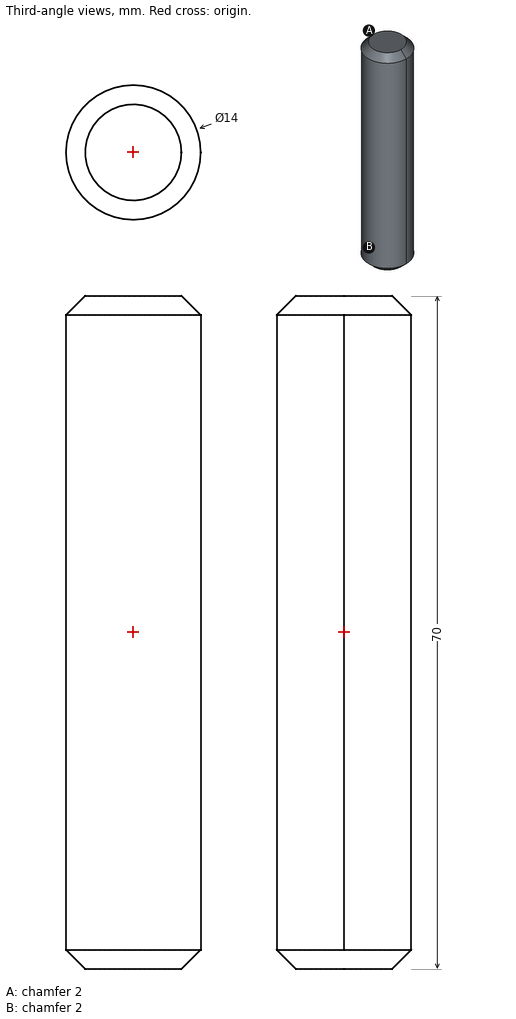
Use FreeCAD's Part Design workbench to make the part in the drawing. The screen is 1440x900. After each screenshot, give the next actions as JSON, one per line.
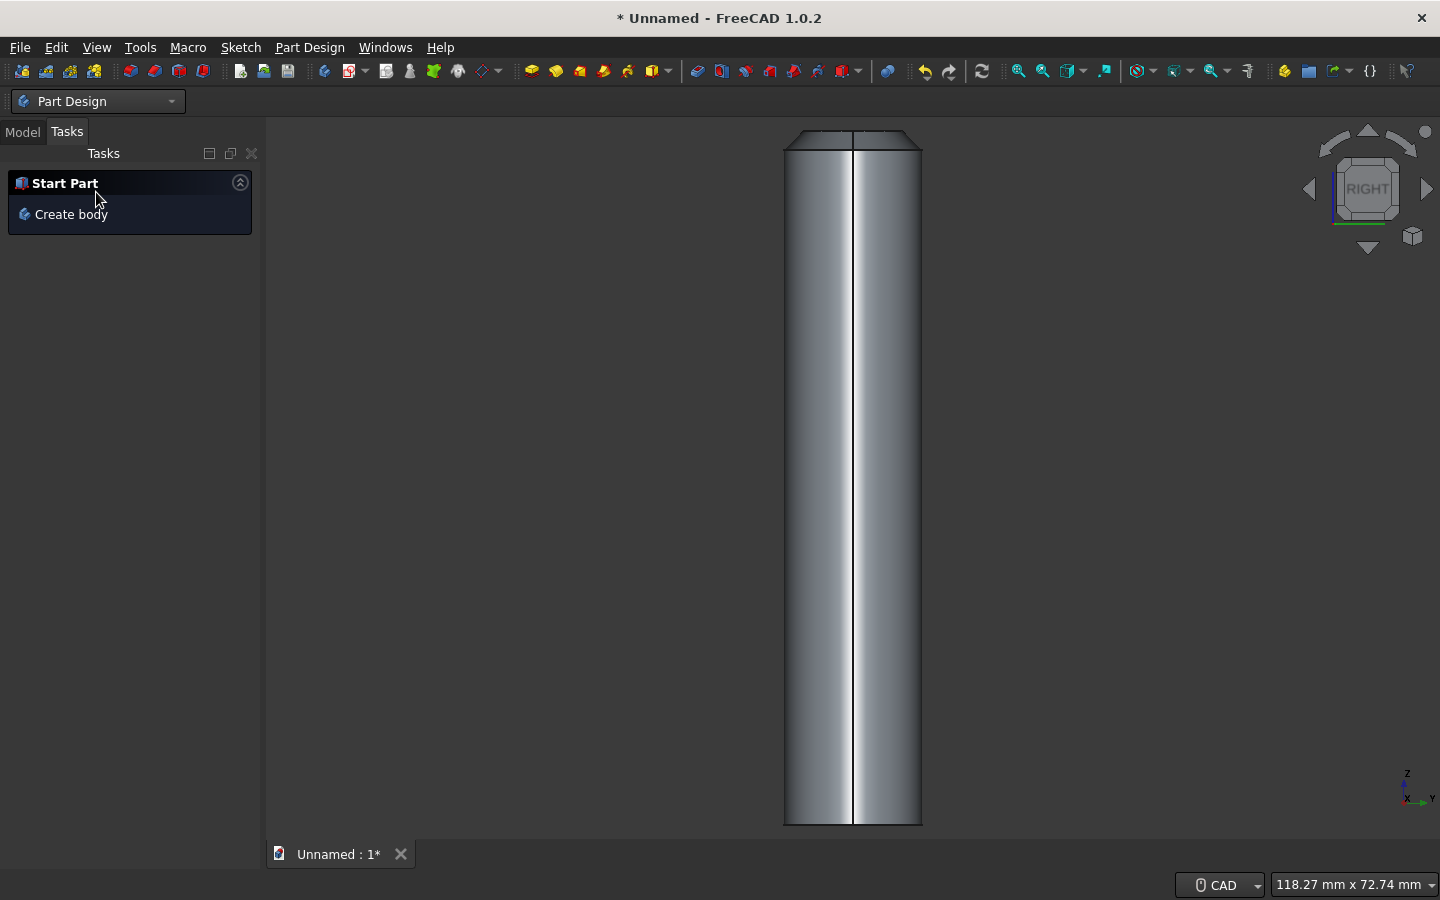
{"action": "key", "text": "5"}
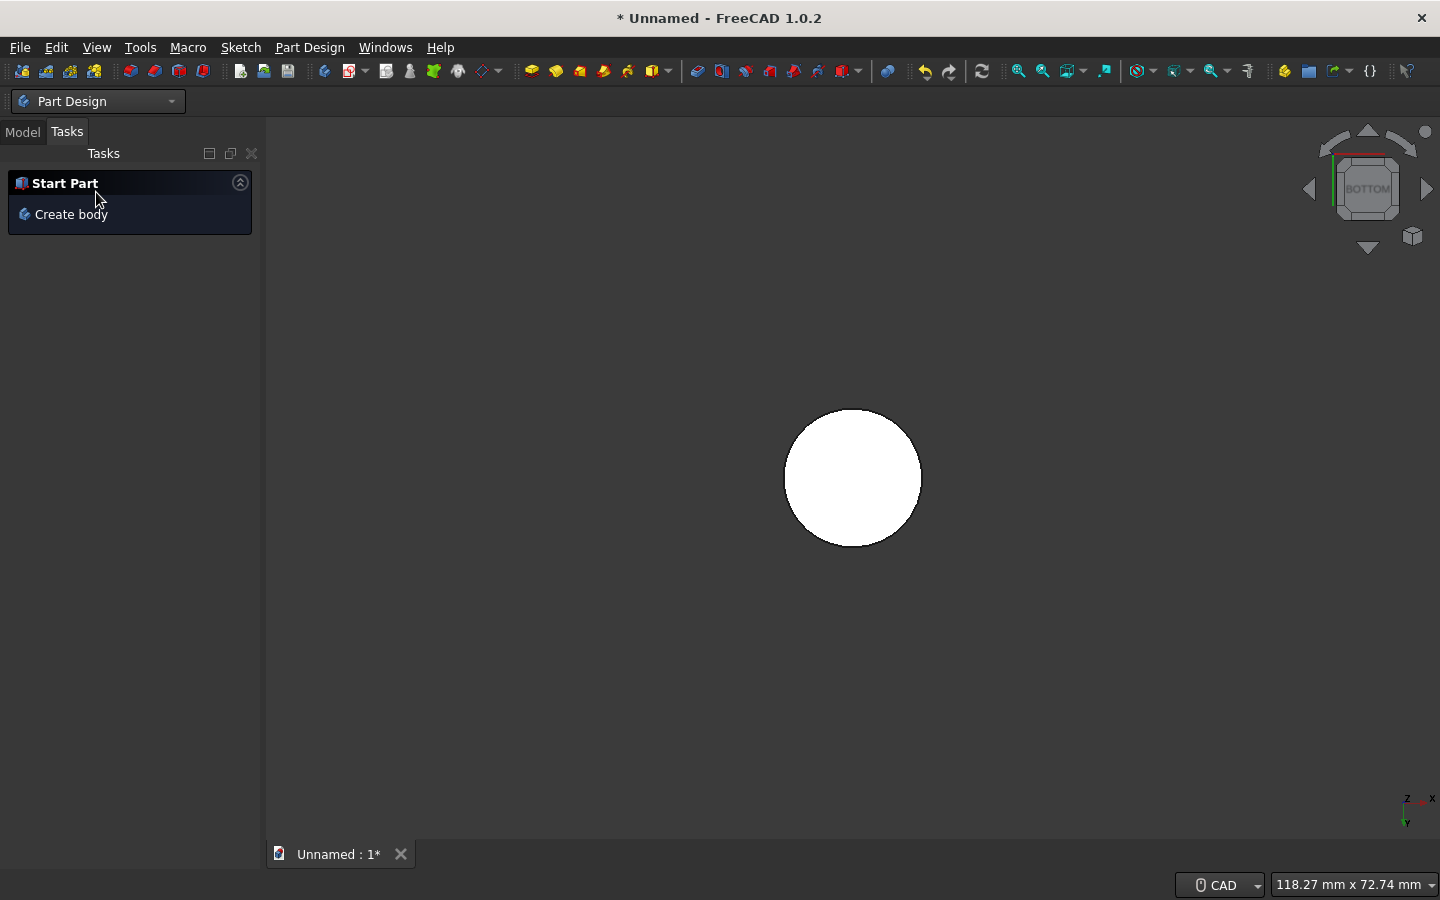
{"action": "key", "text": "v f"}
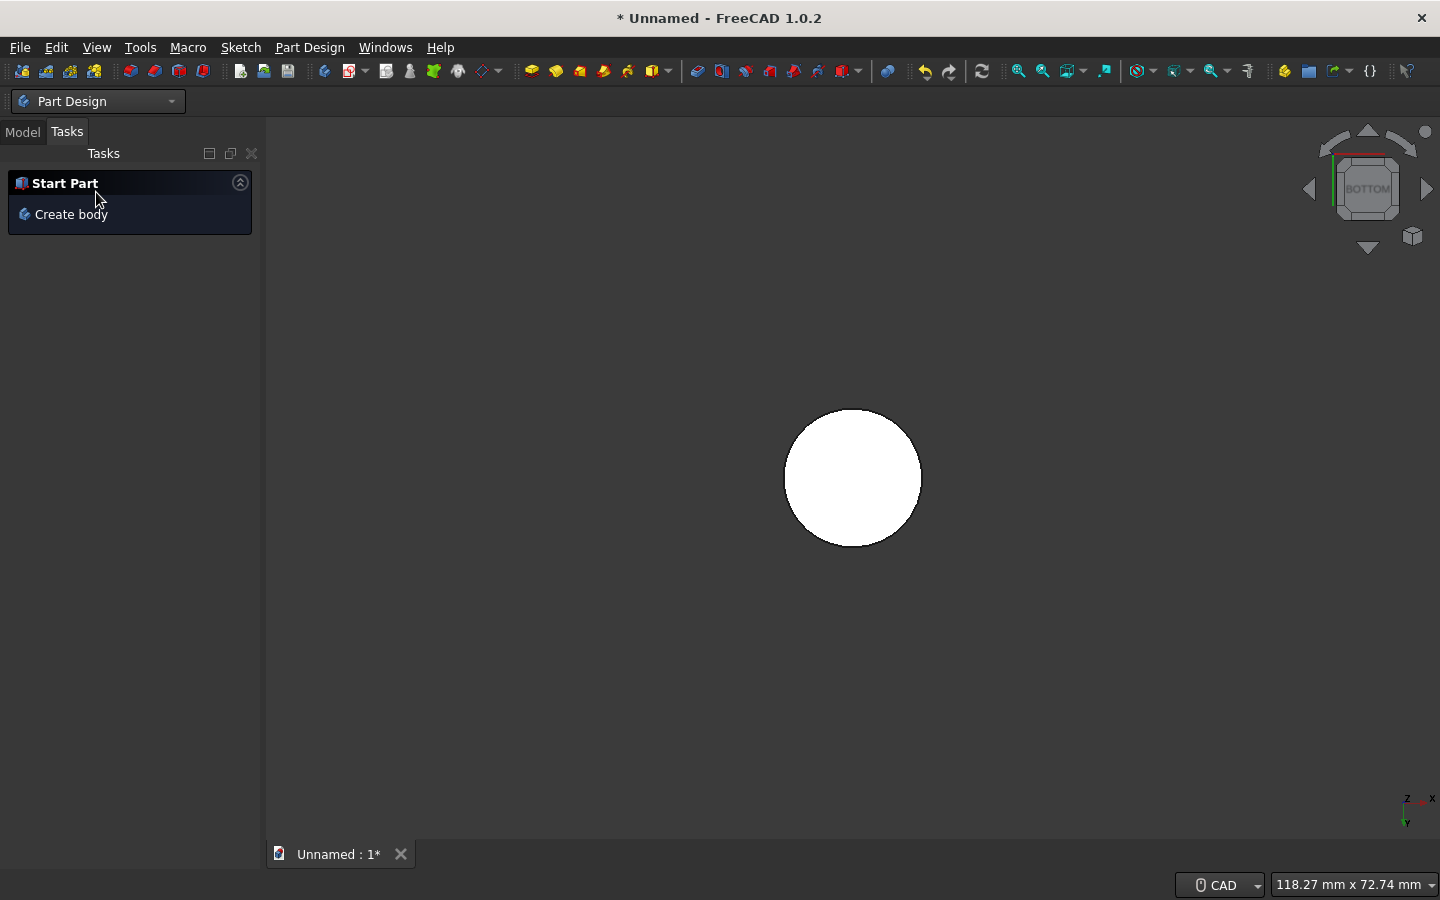
{"action": "left_click", "coordinate": [783, 477]}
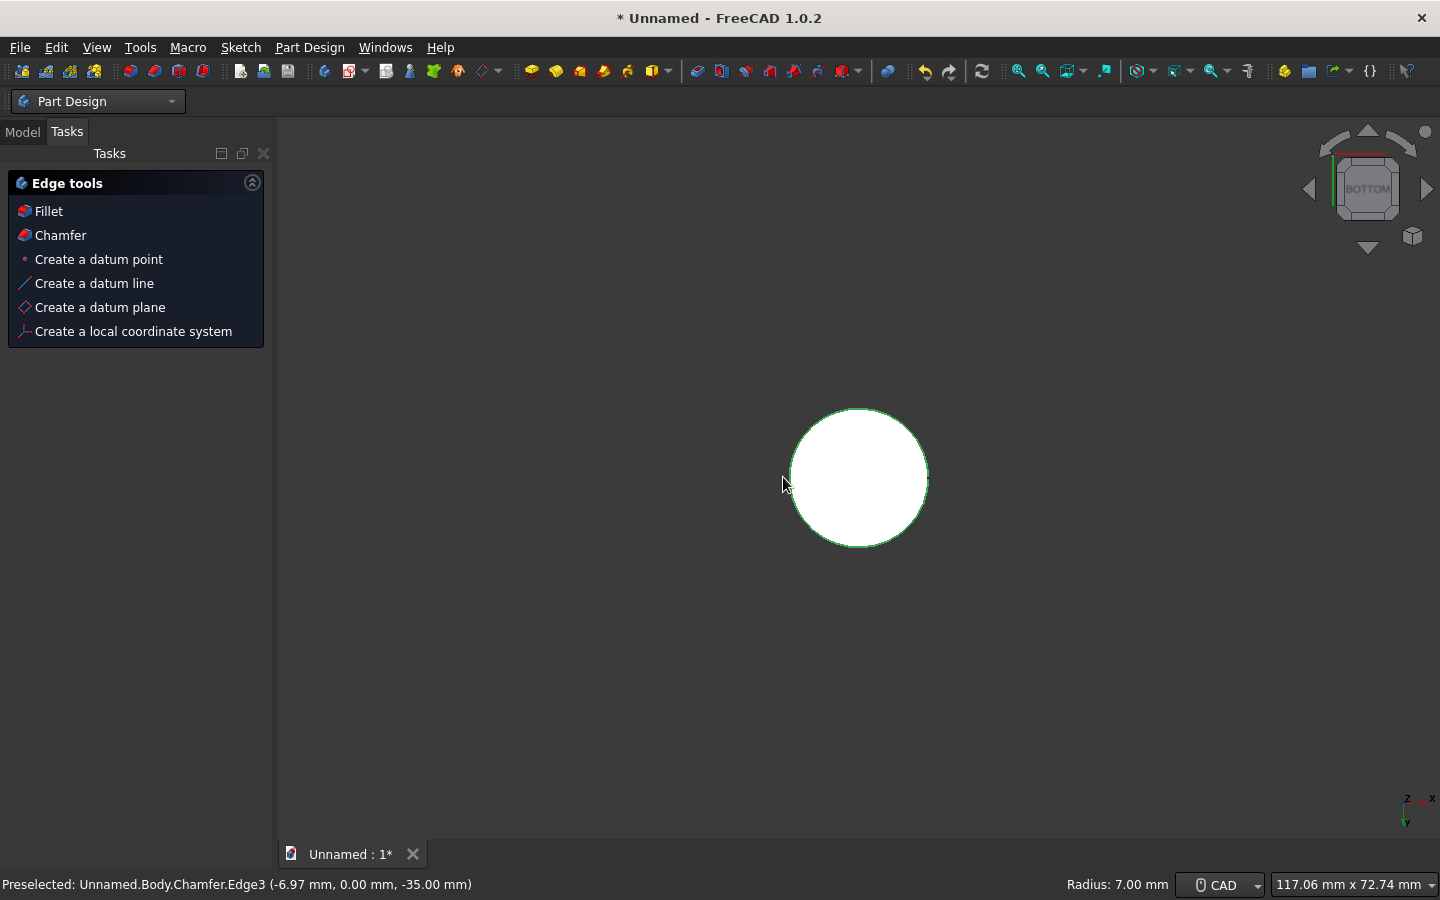
{"action": "left_click", "coordinate": [156, 72]}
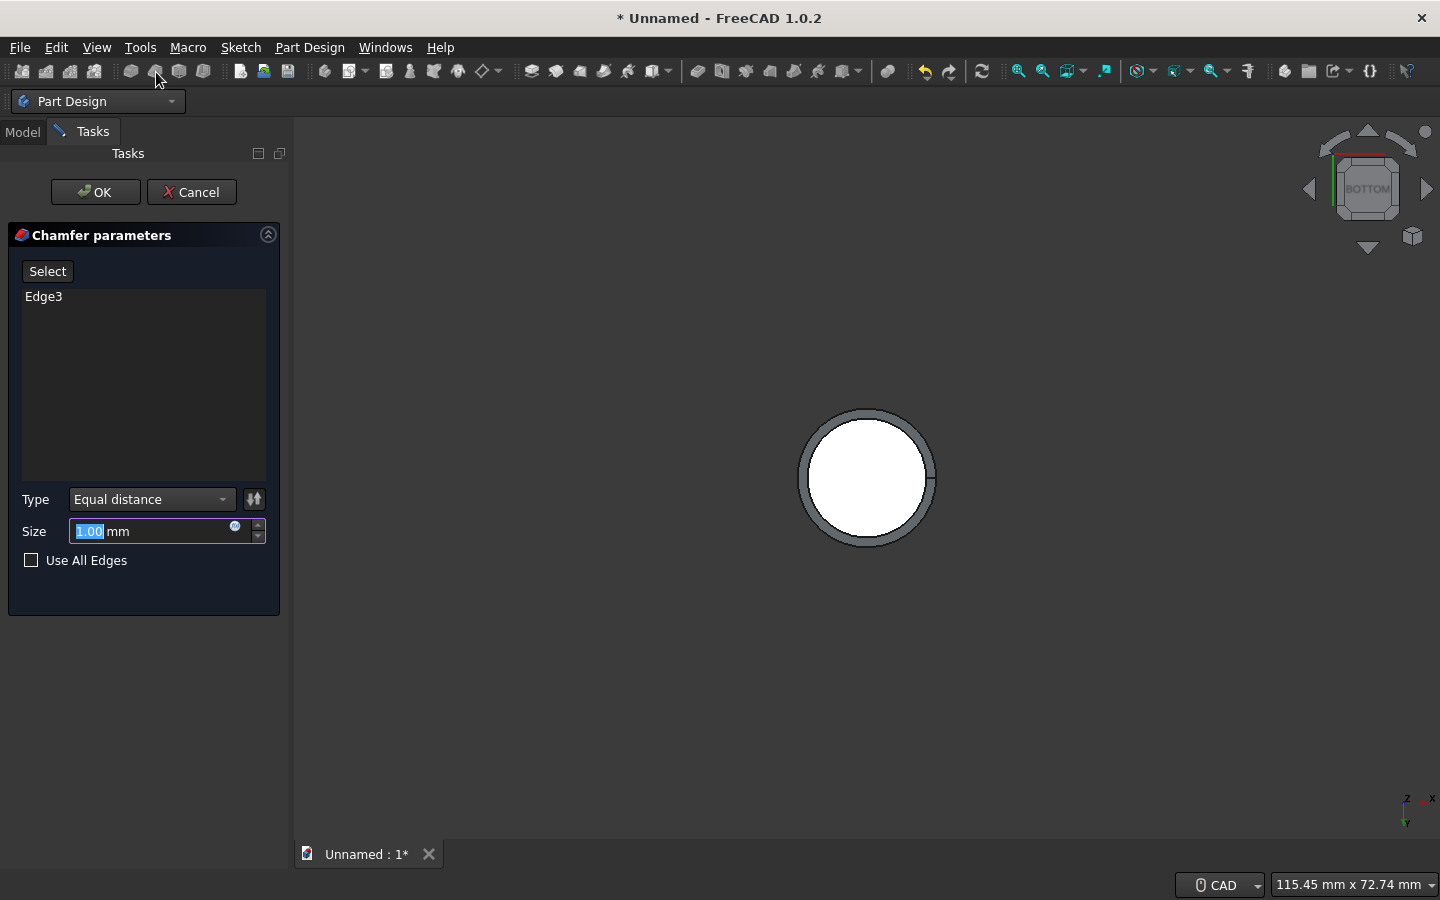
{"action": "type", "text": "2"}
{"action": "key", "text": "Tab"}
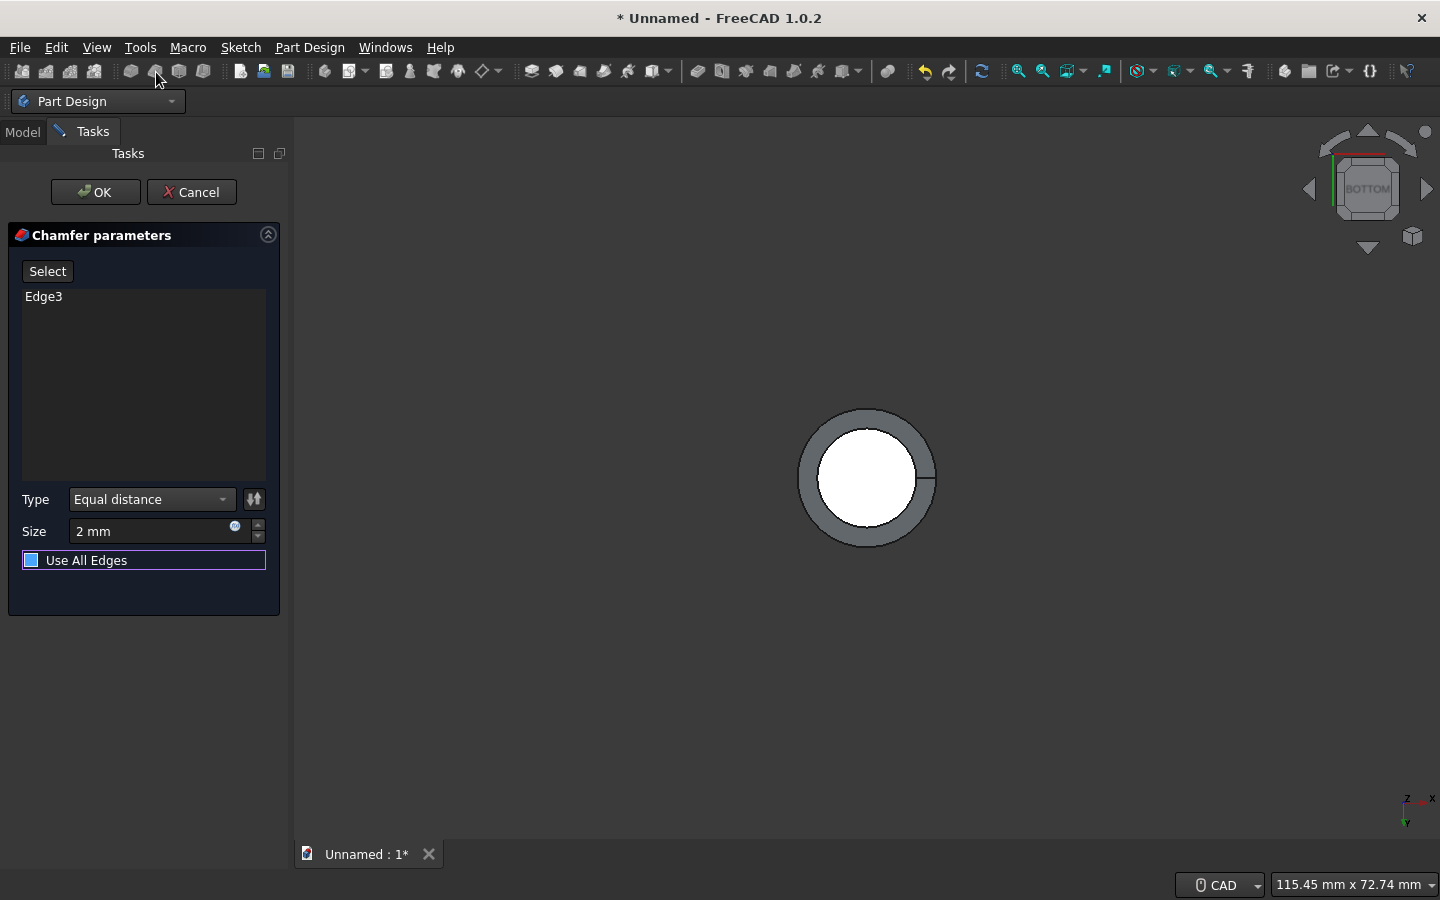
{"action": "left_click", "coordinate": [96, 192]}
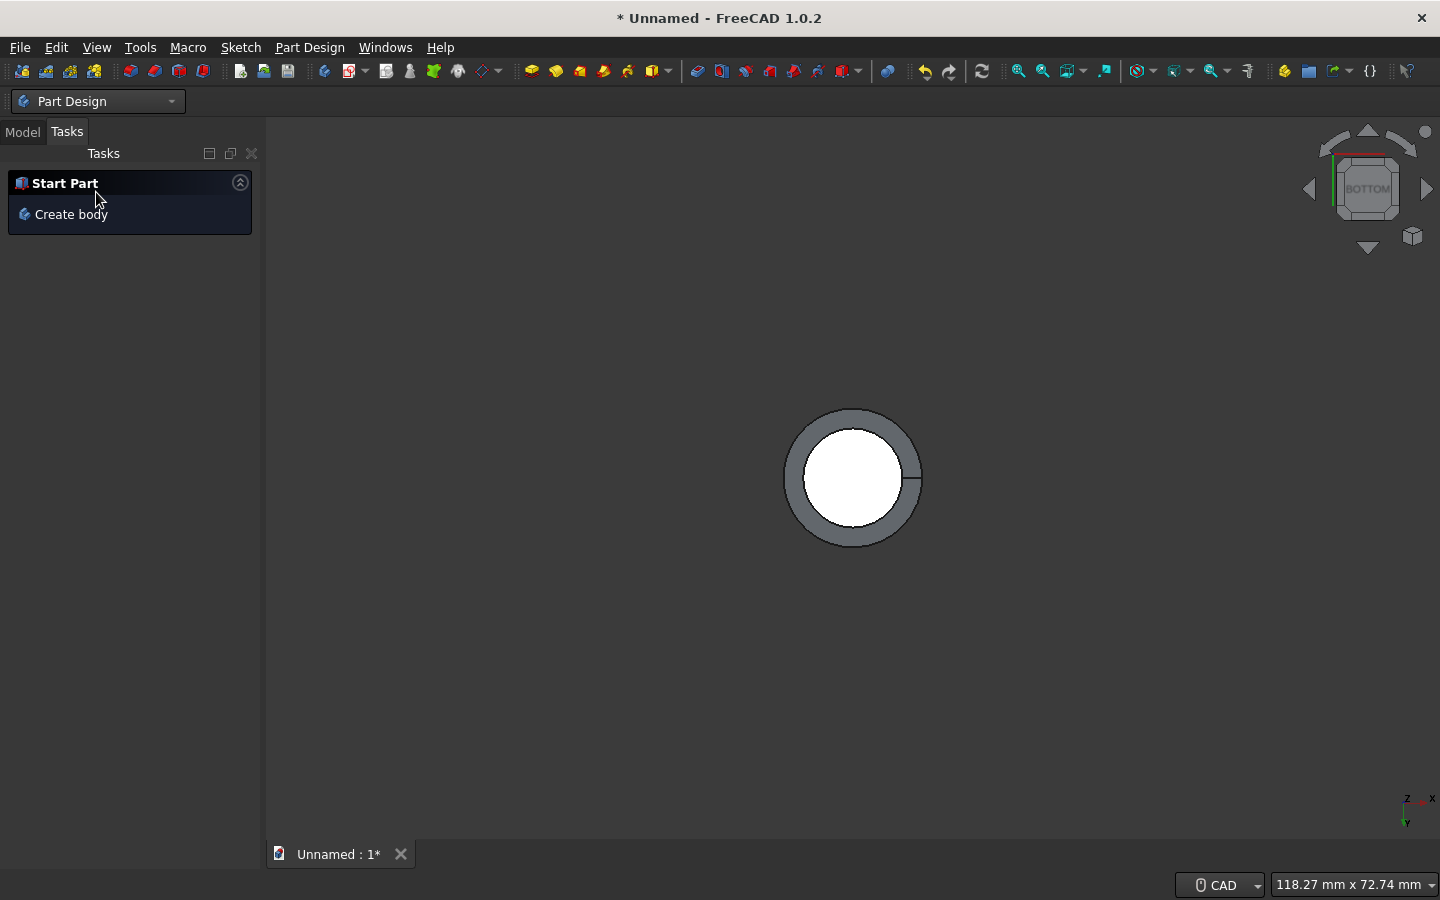
{"action": "key", "text": "0"}